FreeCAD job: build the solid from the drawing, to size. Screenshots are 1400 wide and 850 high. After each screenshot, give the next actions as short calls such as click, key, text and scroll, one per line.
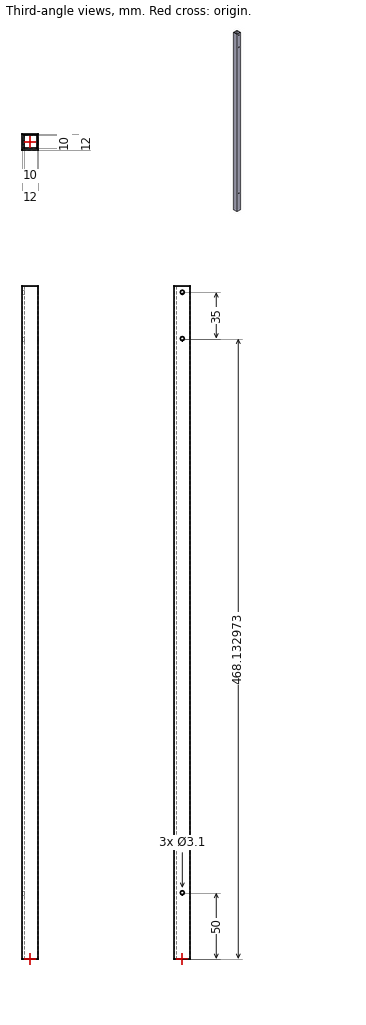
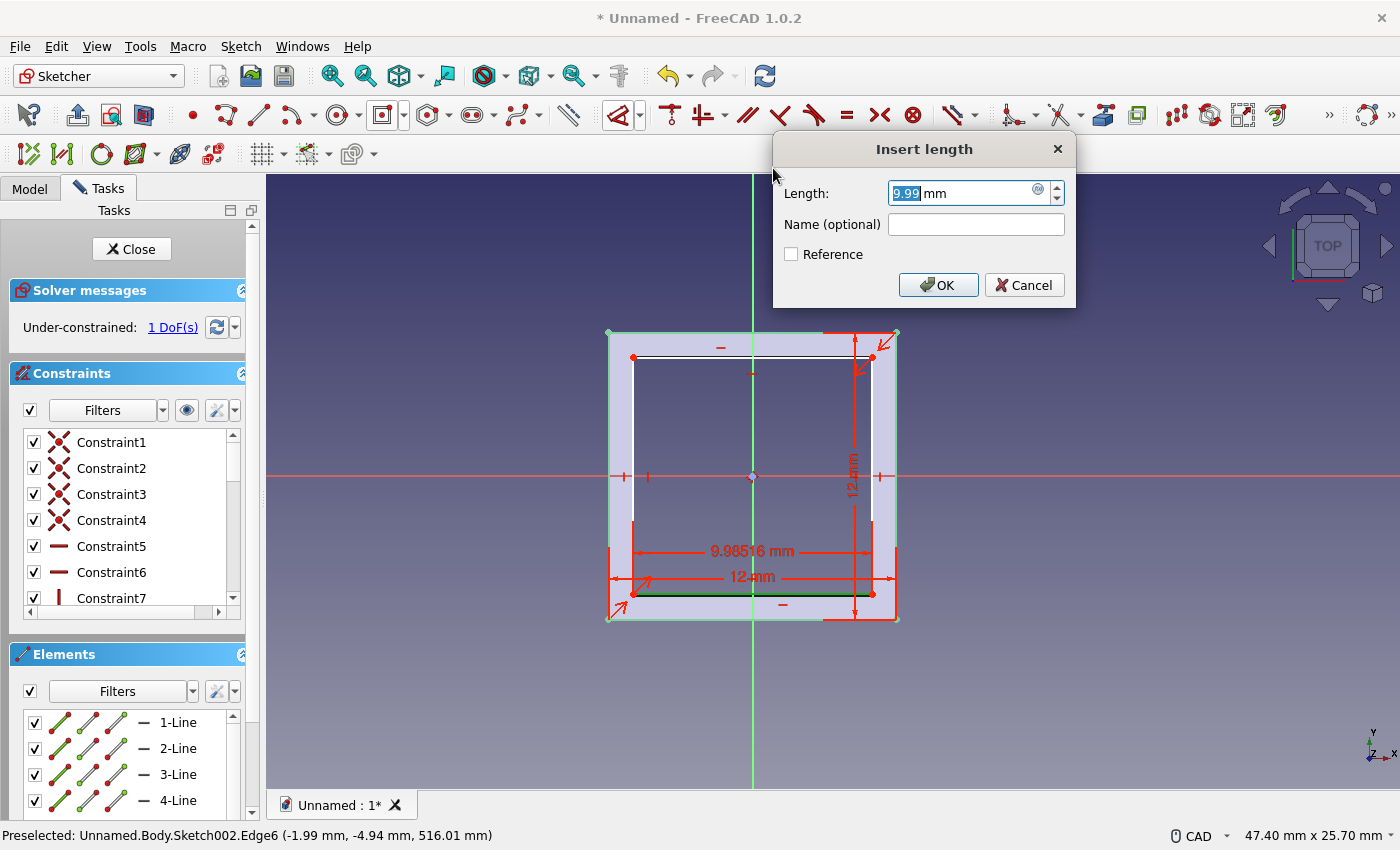
text(10)
key(Return)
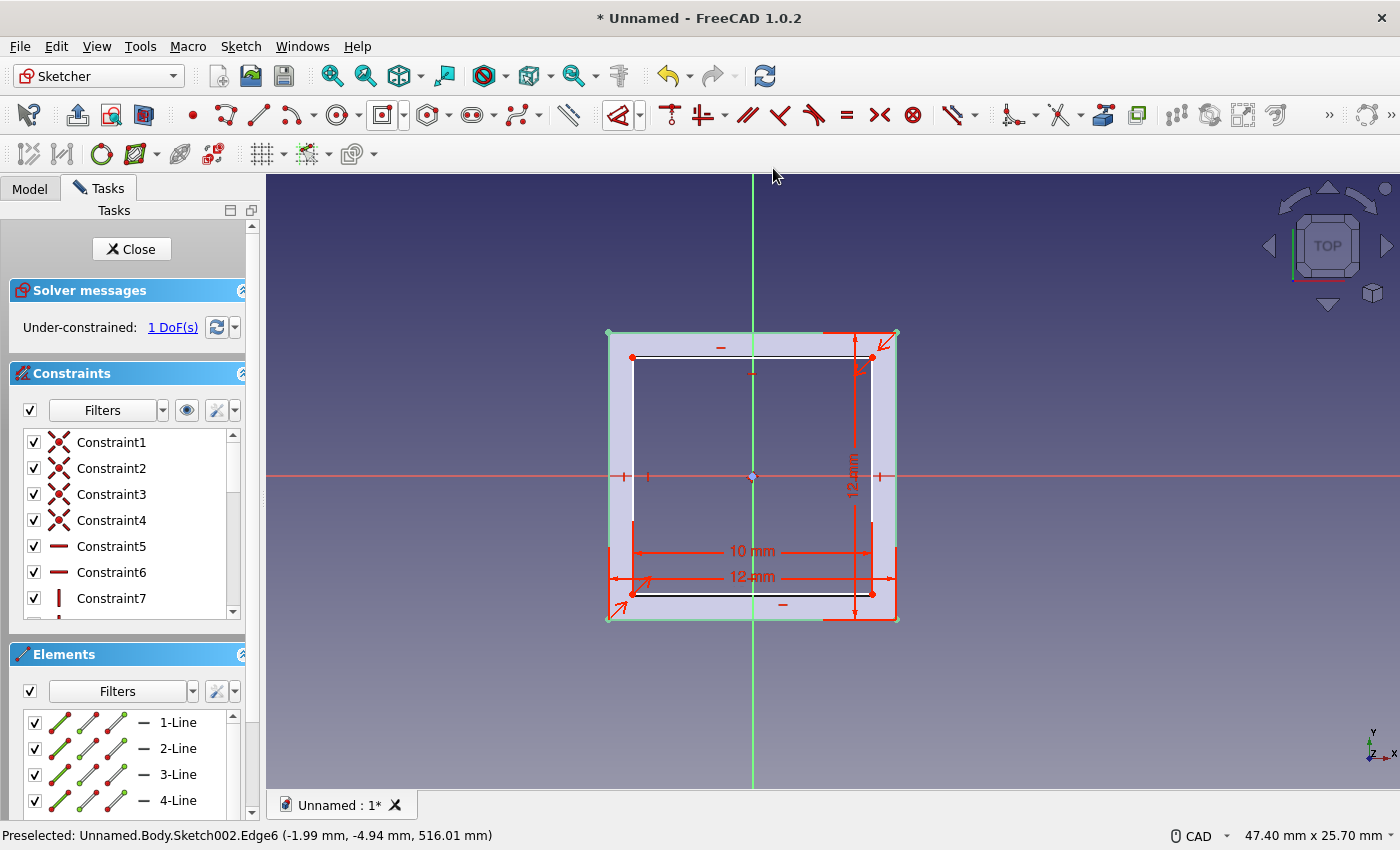
click(872, 523)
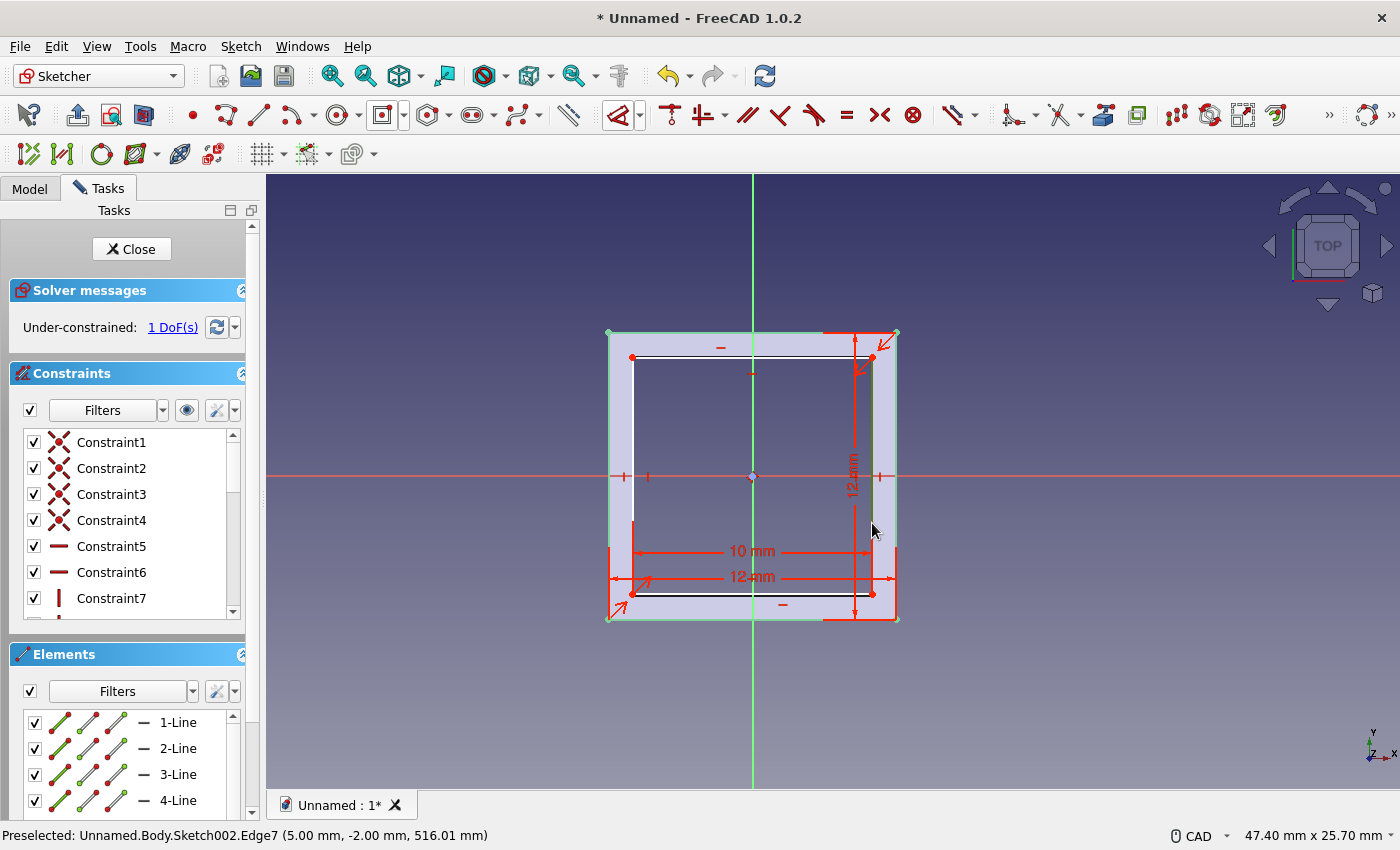
click(640, 116)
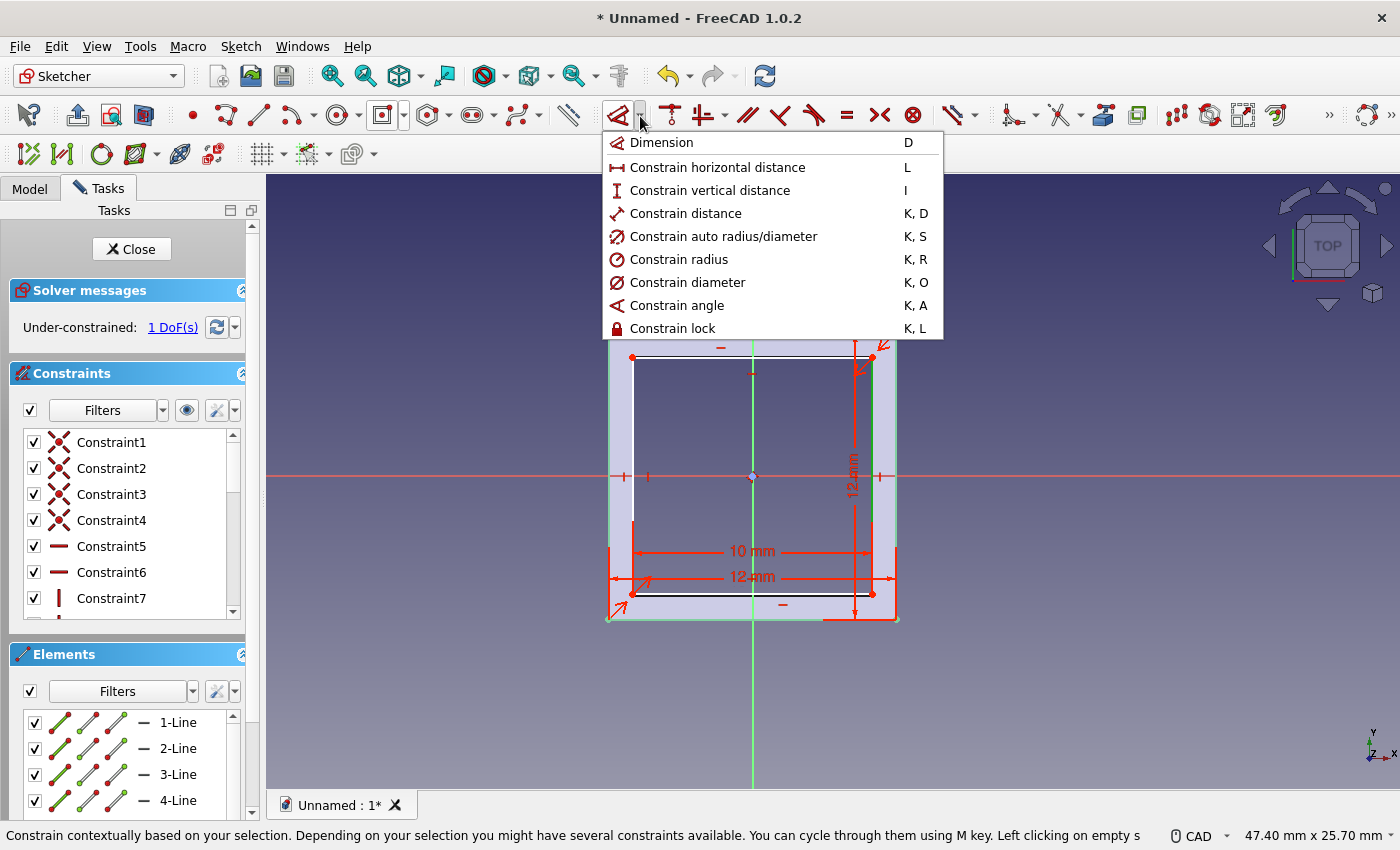
click(773, 190)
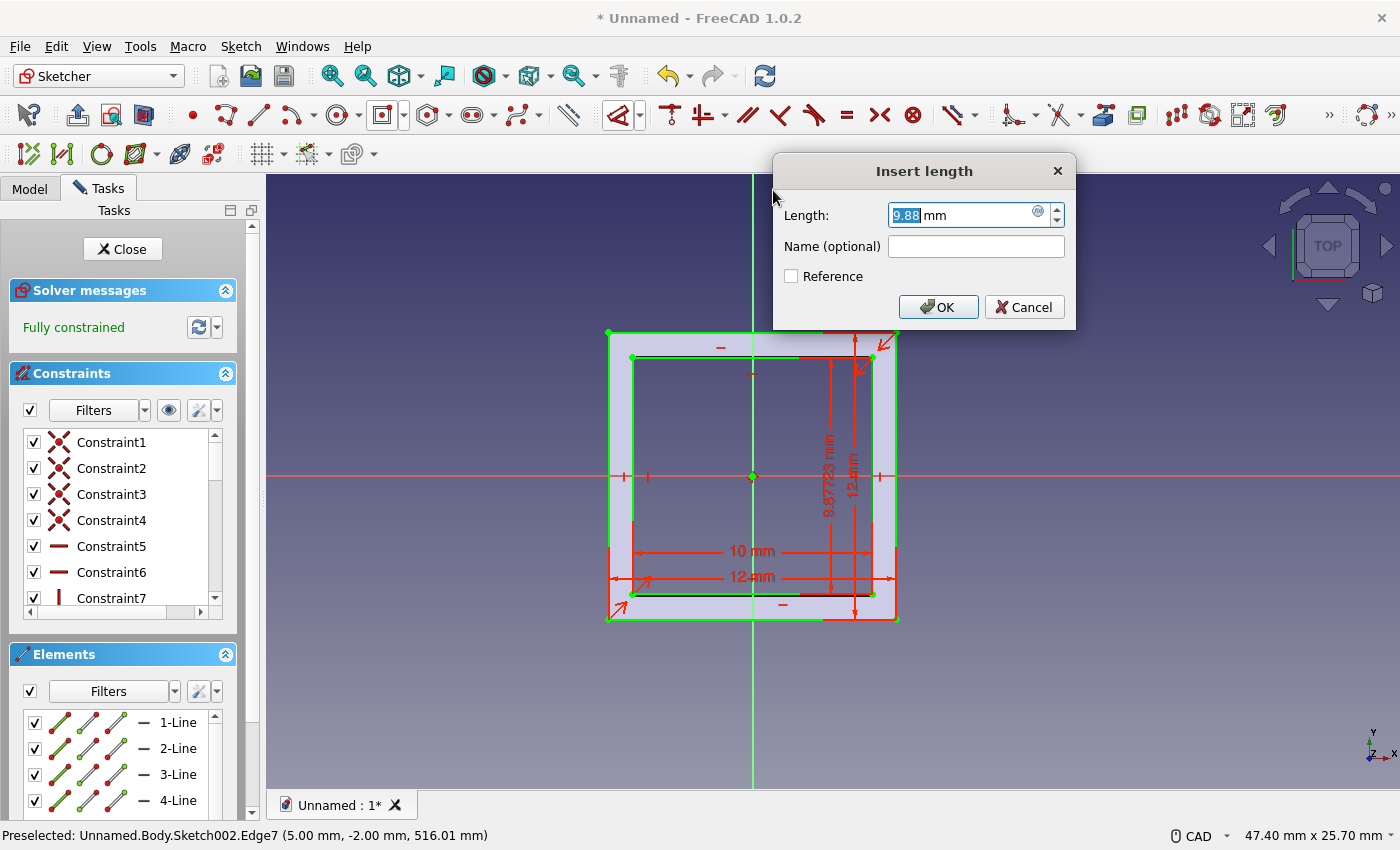
text(10)
key(Return)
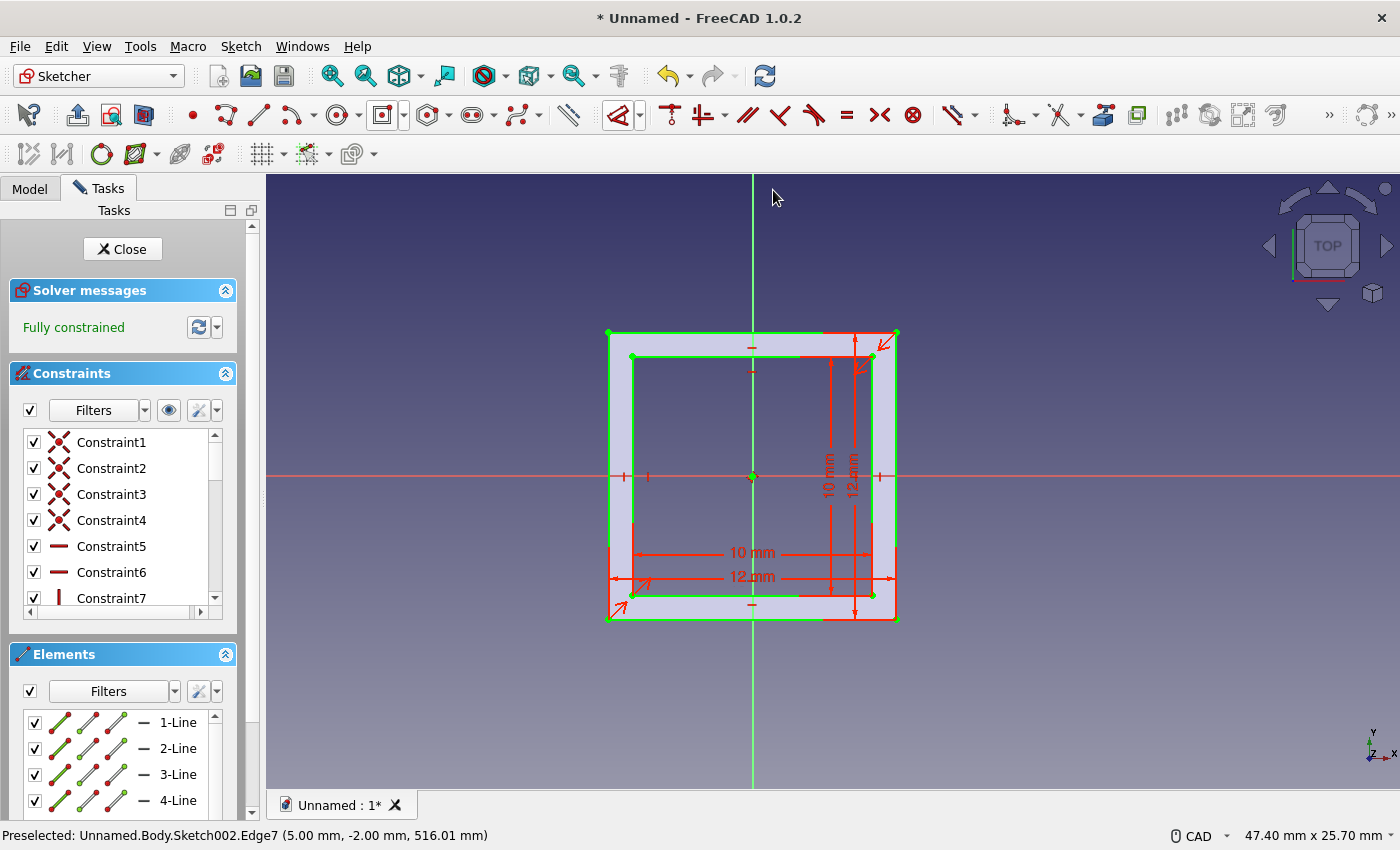
click(123, 249)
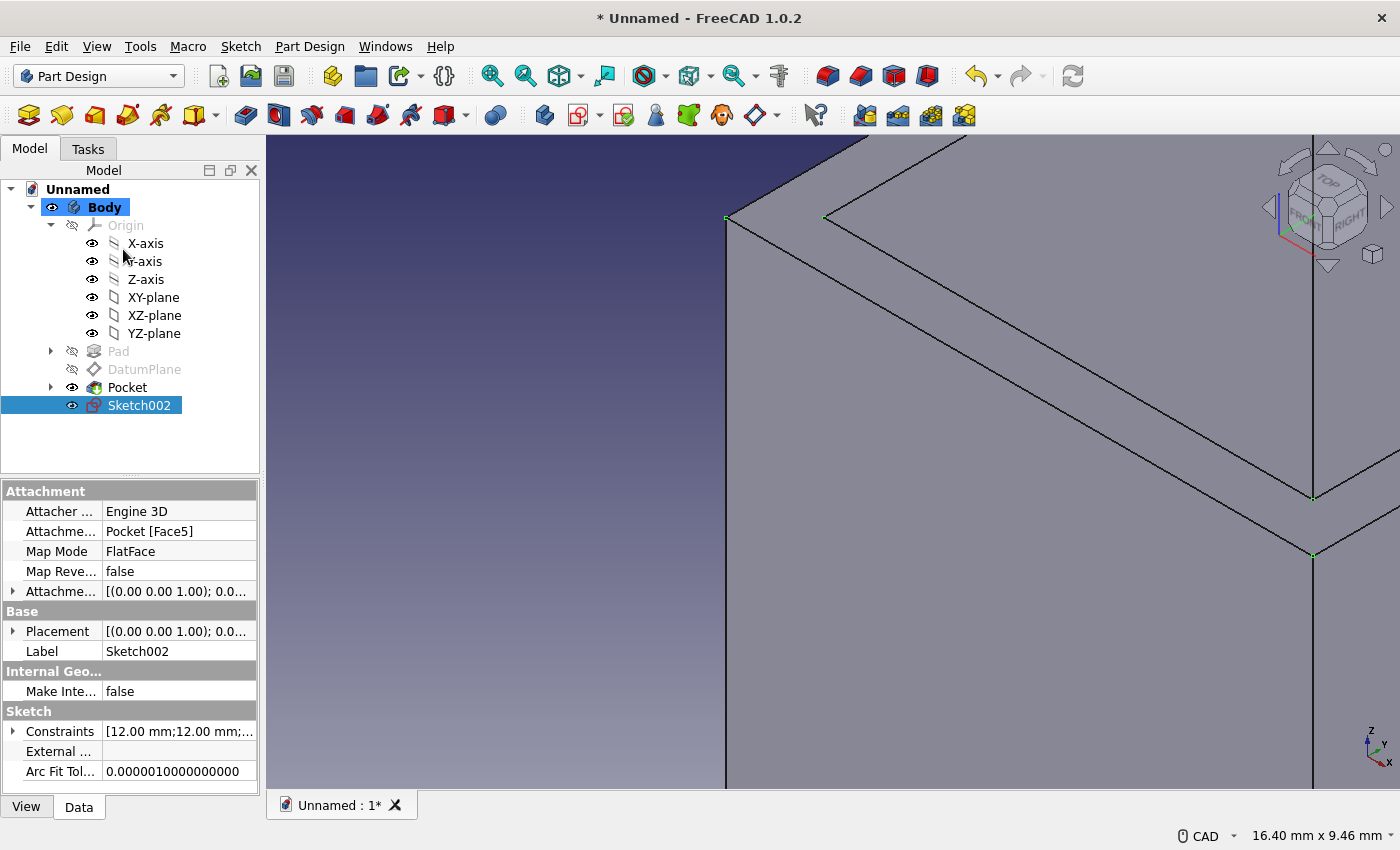
click(246, 116)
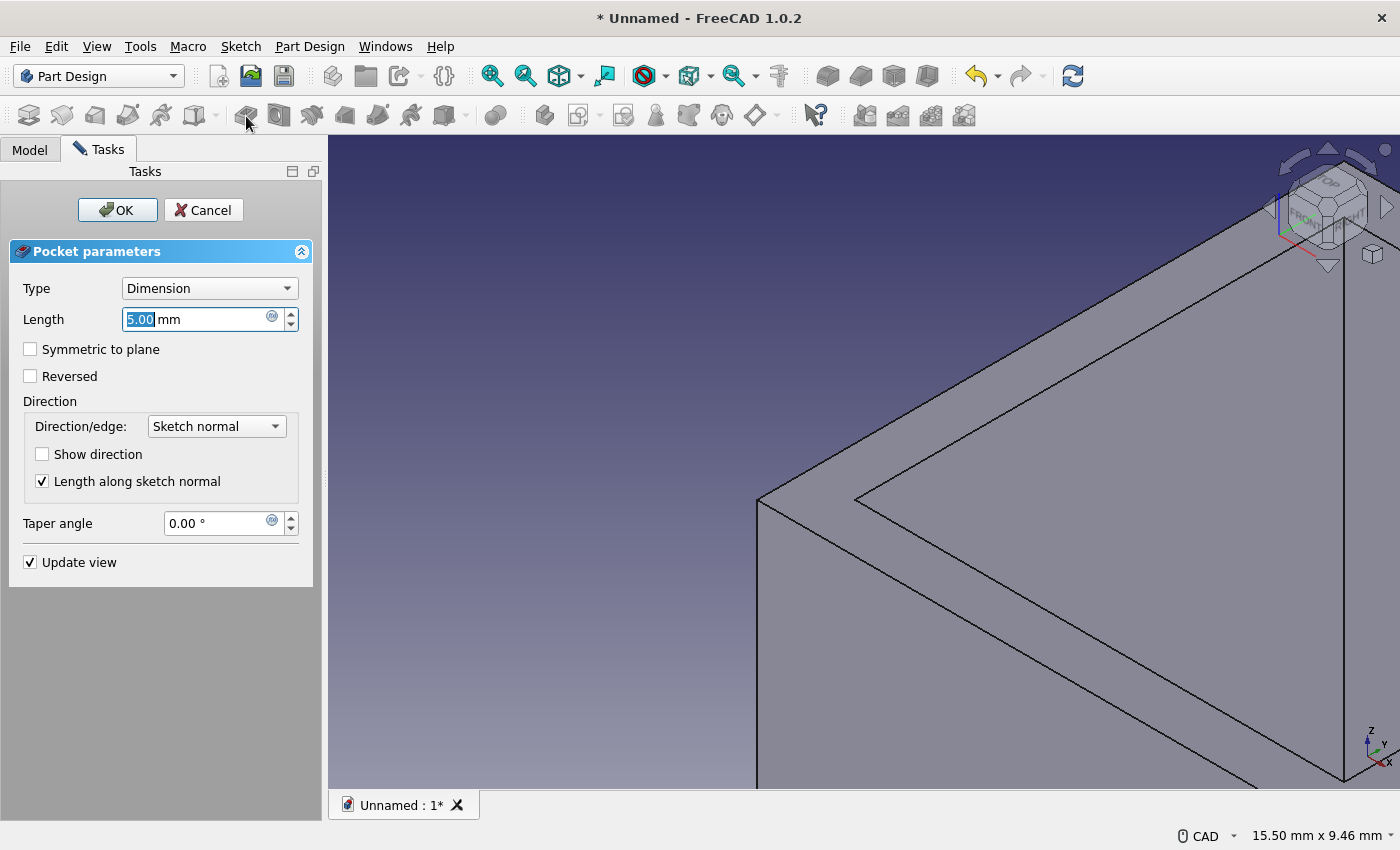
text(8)
key(Tab)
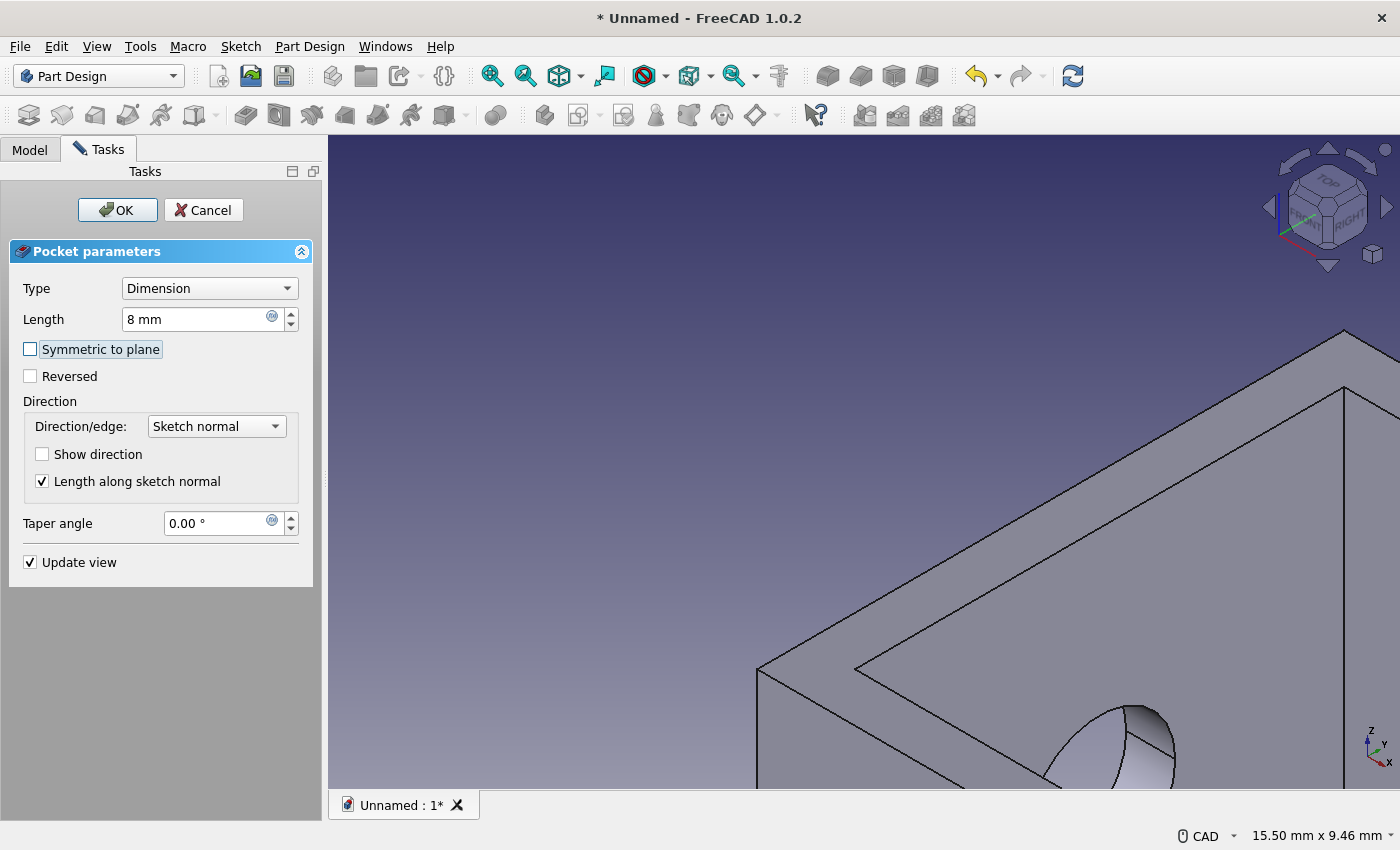
click(118, 210)